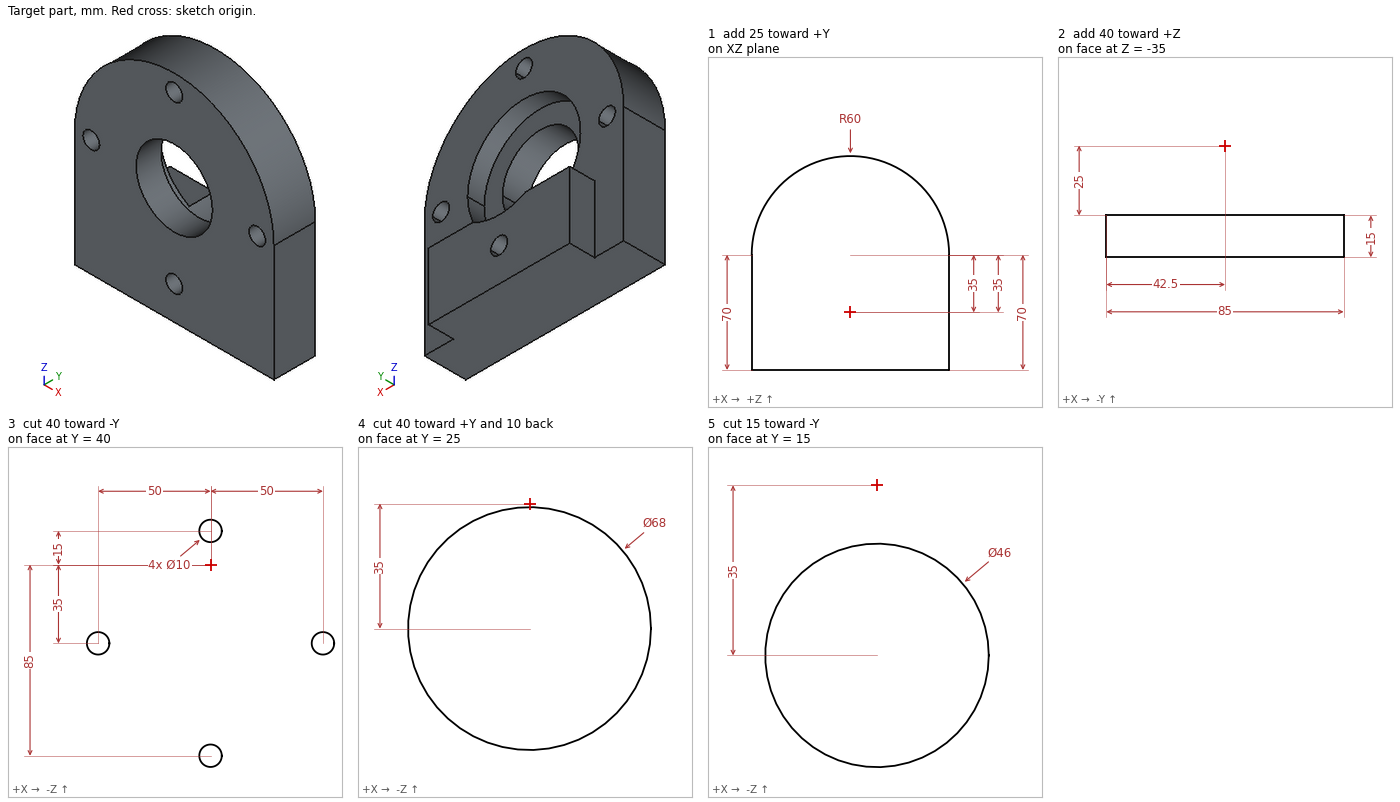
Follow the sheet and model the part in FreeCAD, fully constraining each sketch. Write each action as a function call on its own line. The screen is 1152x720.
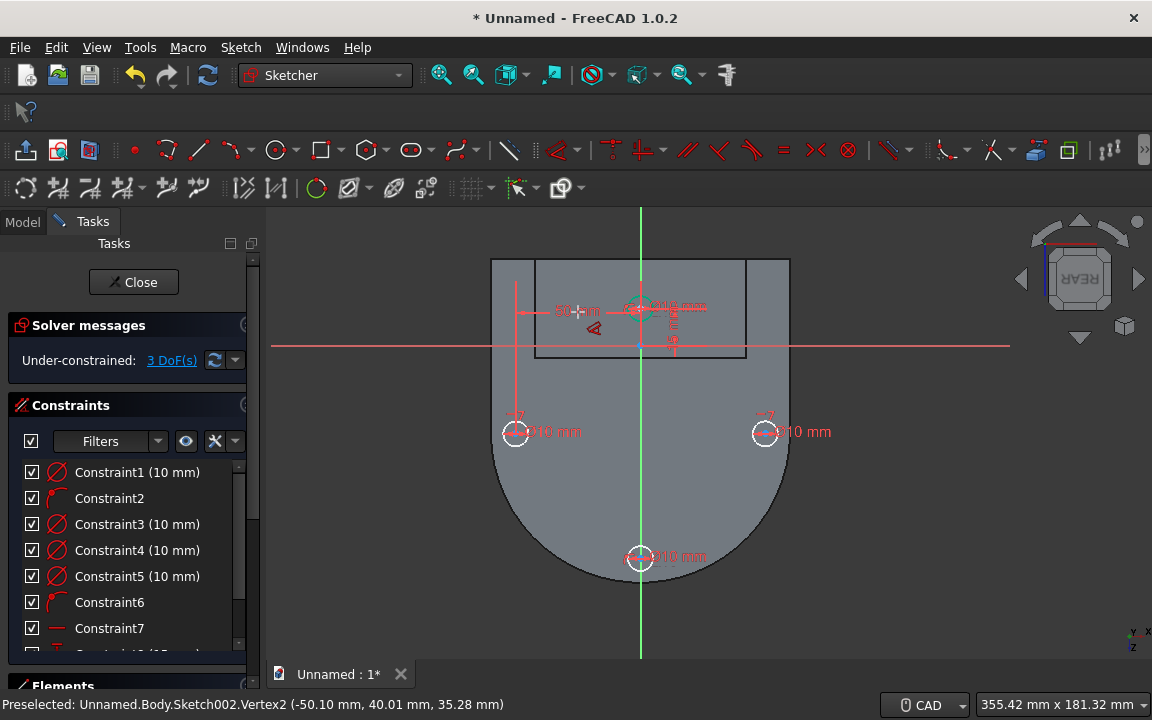
click(516, 434)
click(482, 390)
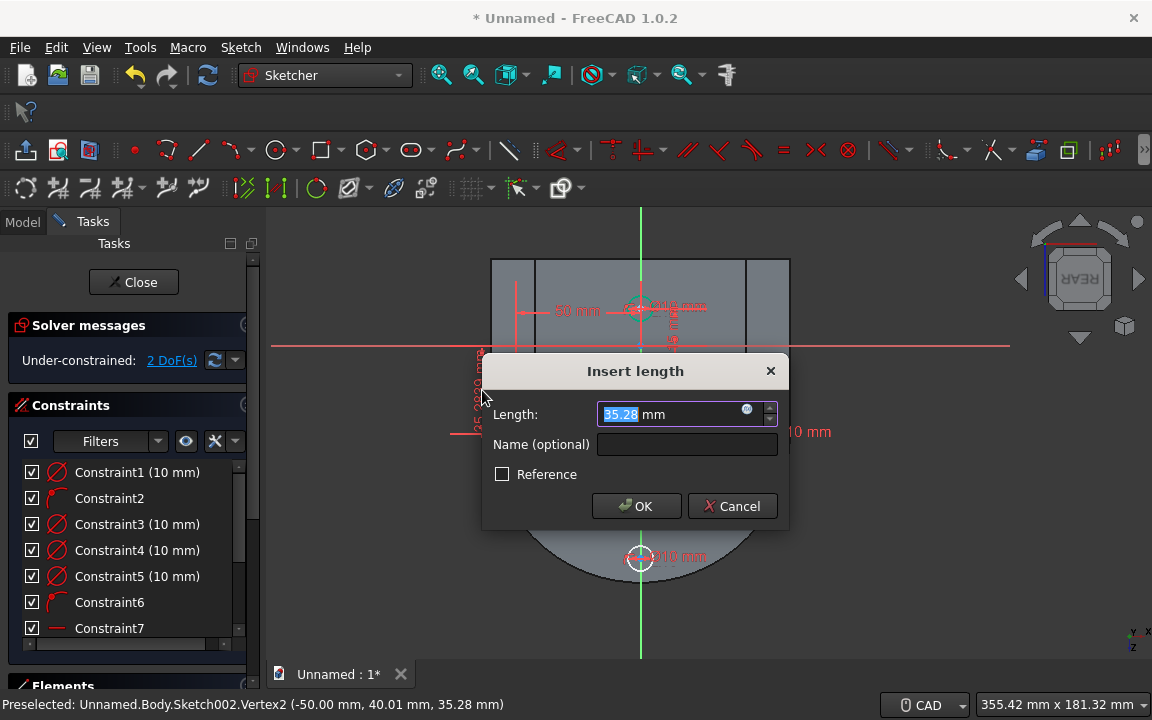
text(35)
key(Return)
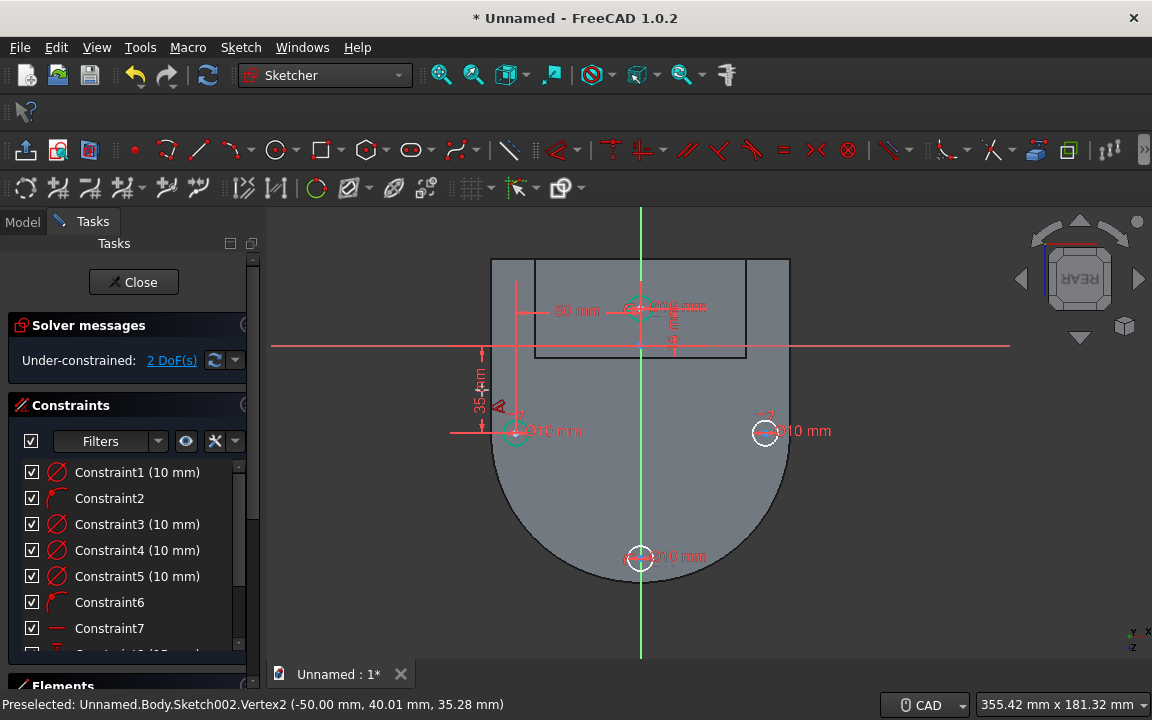
click(765, 433)
click(747, 312)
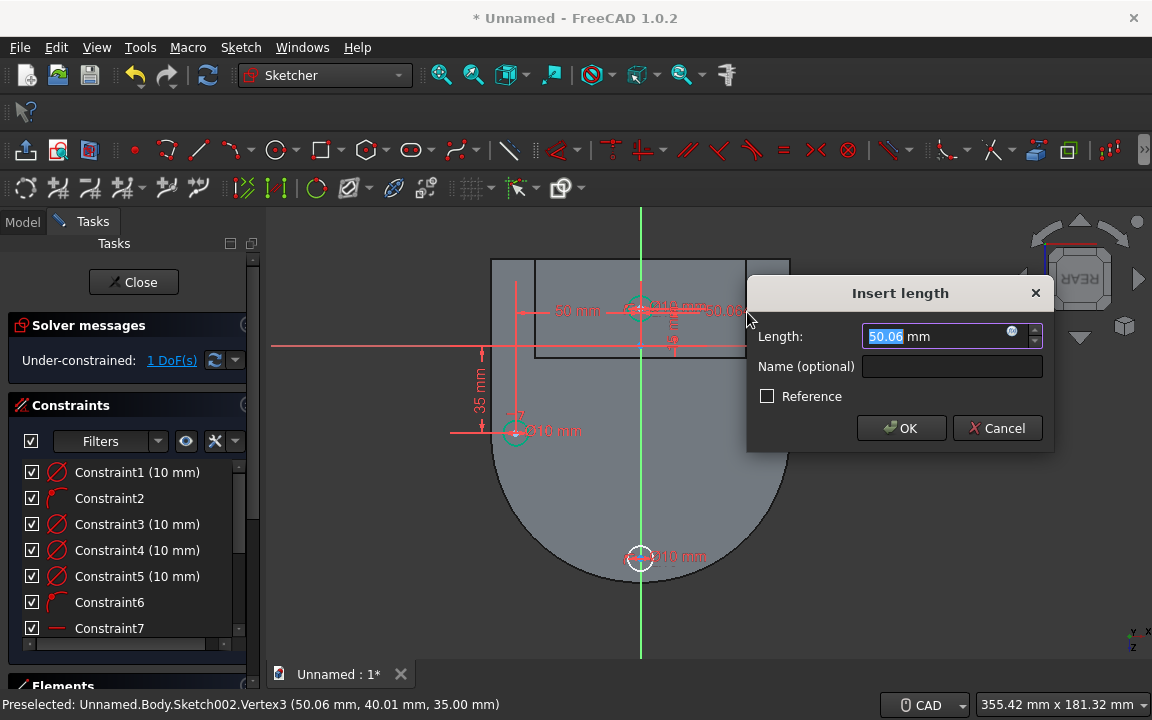
text(50)
key(Return)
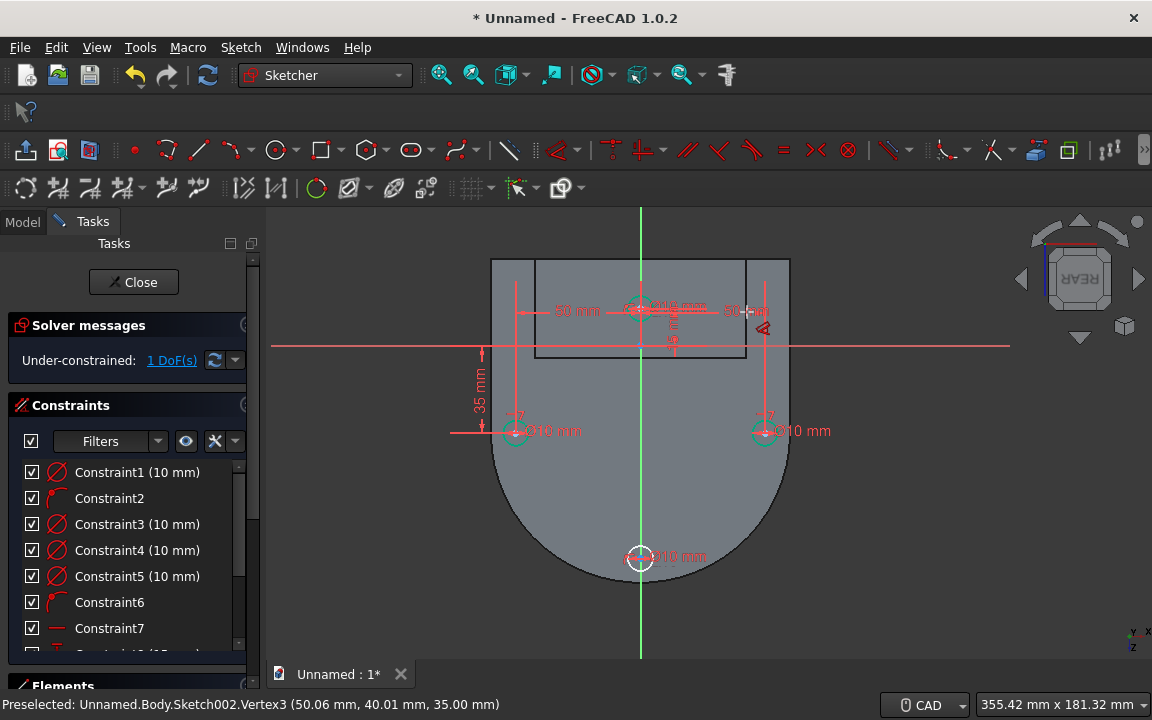
click(641, 559)
click(675, 452)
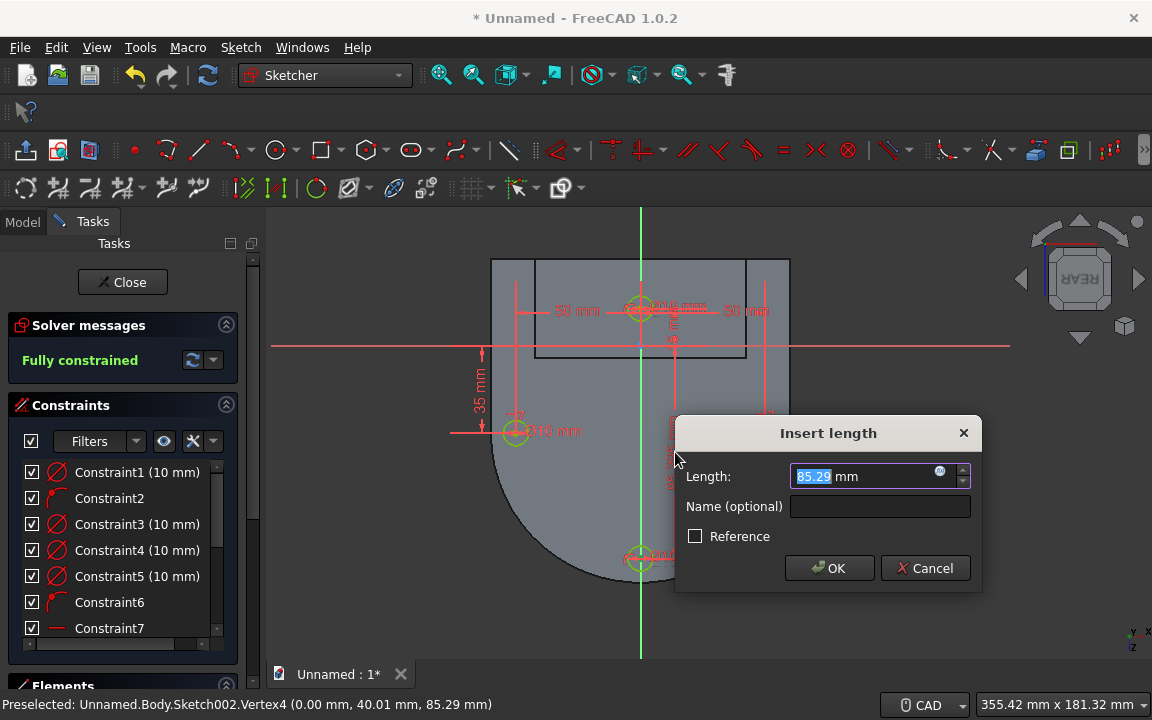
text(85)
key(Return)
key(Escape)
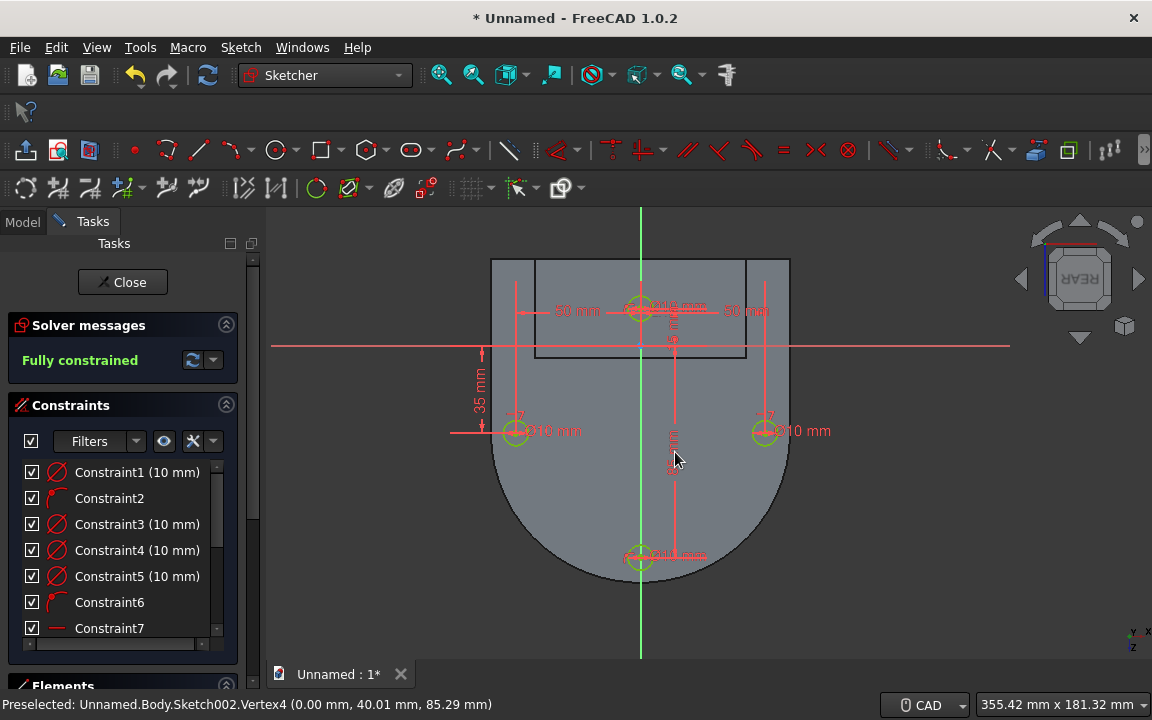
click(123, 282)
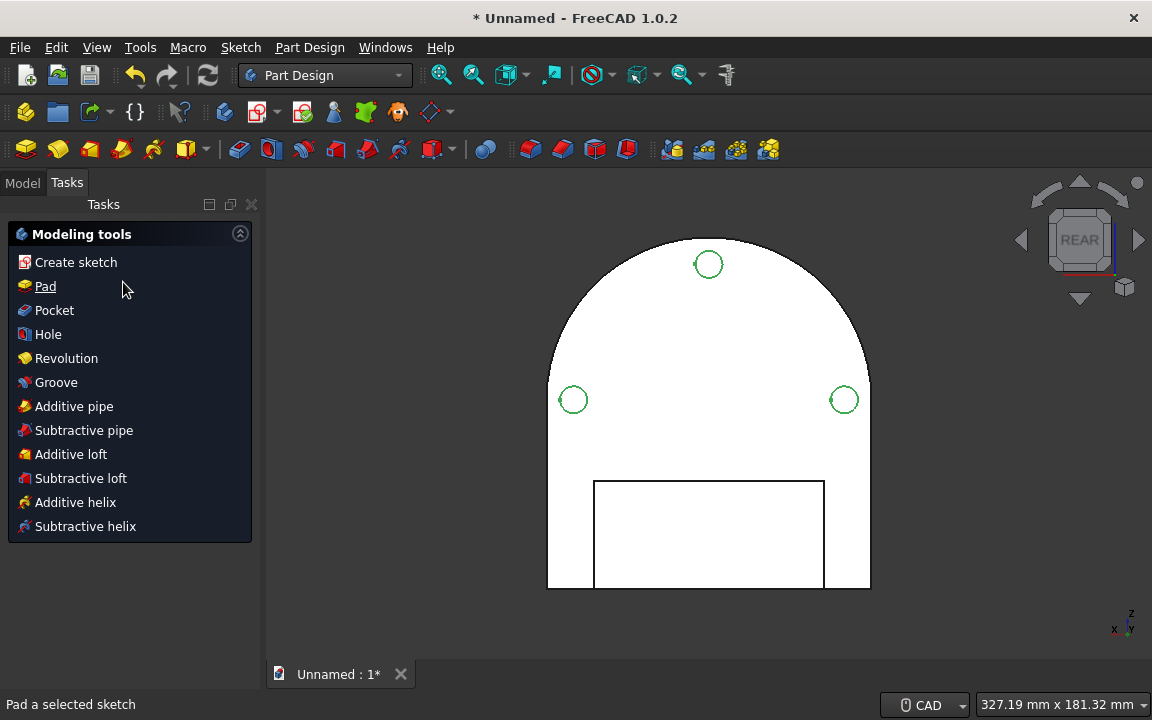
click(240, 150)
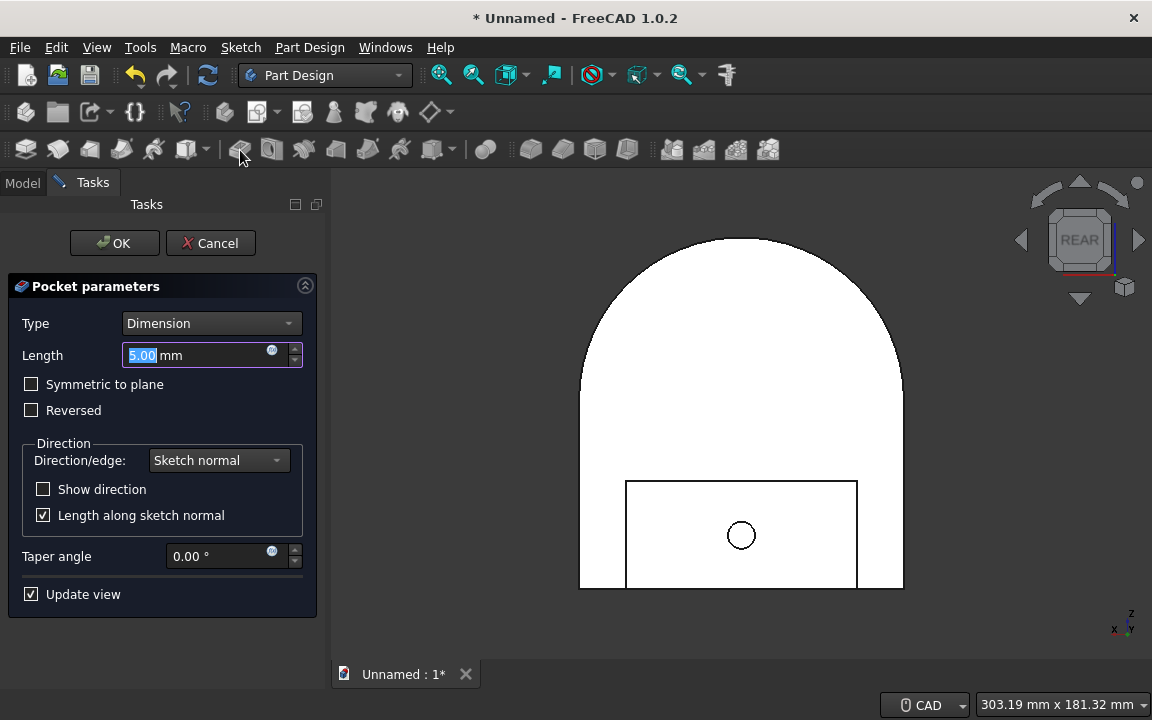
text(40)
key(Tab)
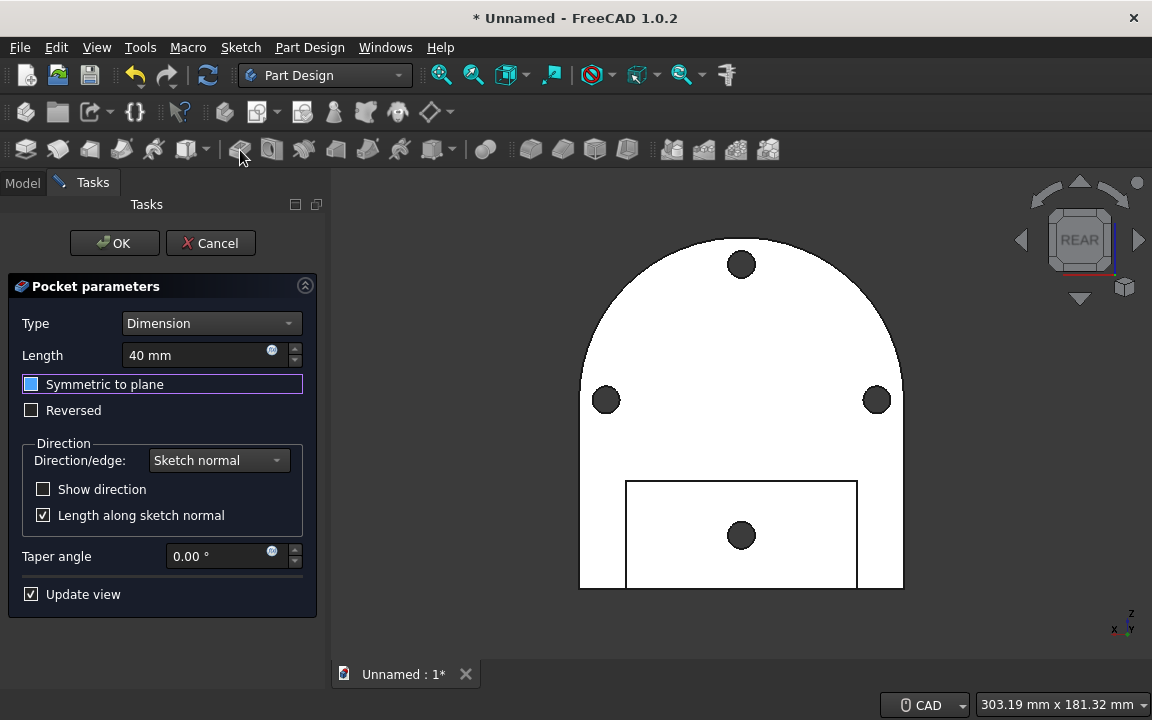
click(115, 243)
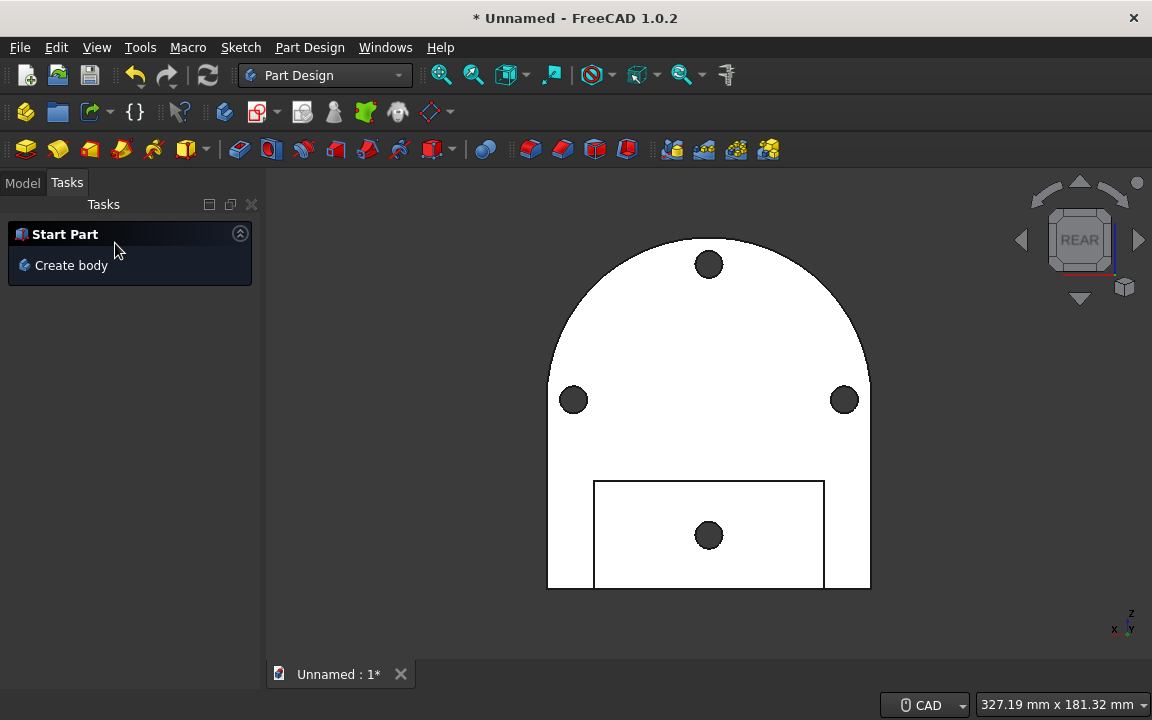
click(709, 362)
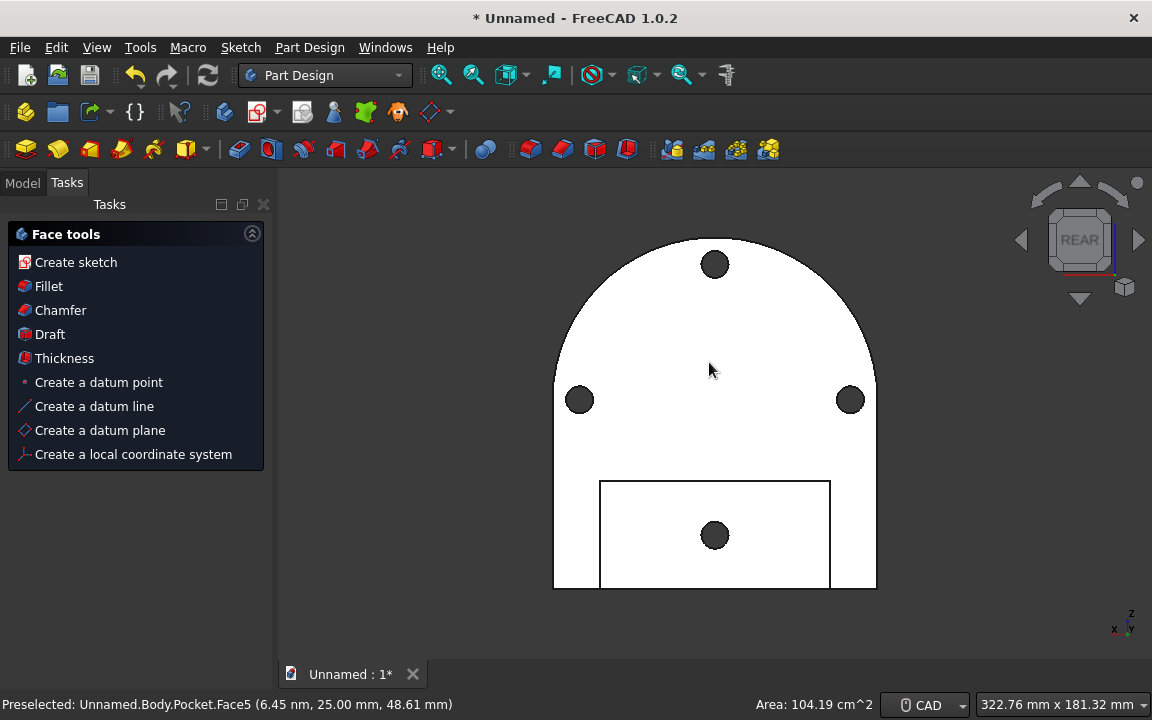
click(258, 112)